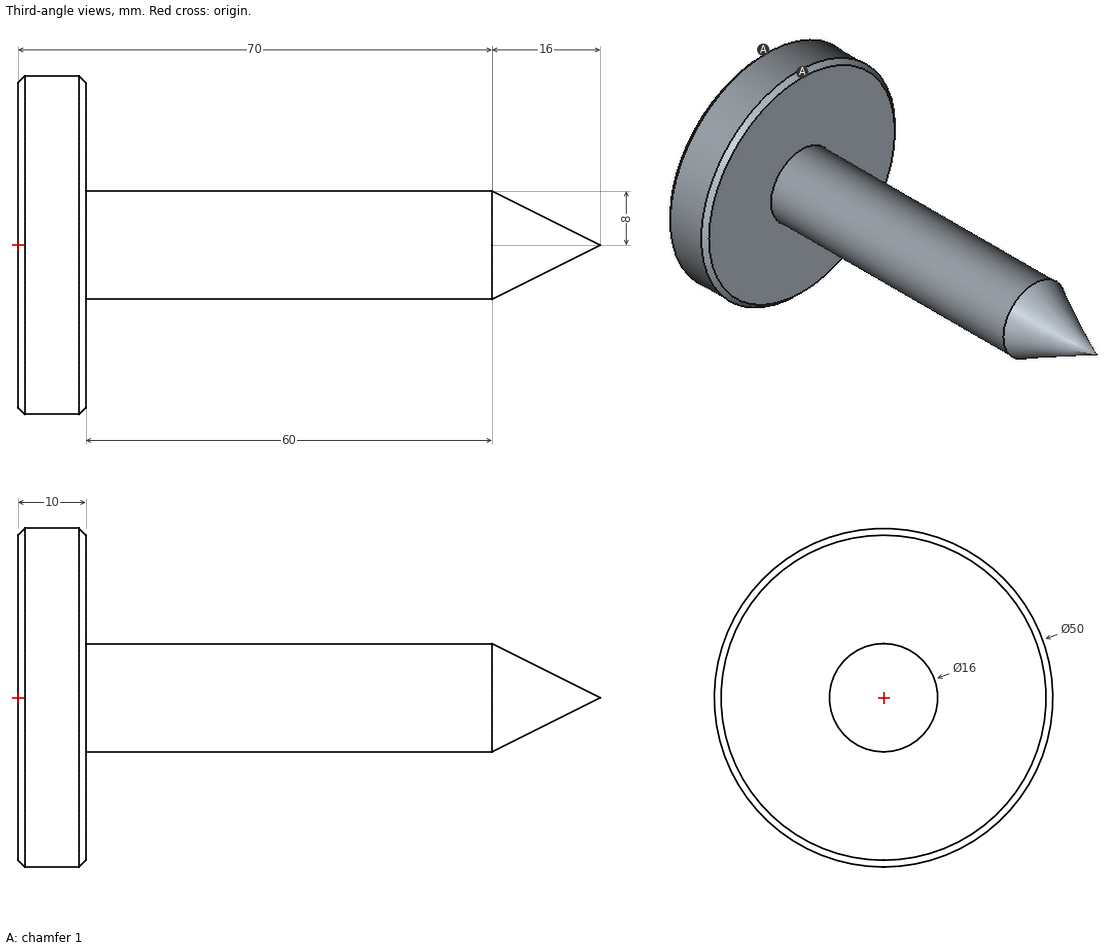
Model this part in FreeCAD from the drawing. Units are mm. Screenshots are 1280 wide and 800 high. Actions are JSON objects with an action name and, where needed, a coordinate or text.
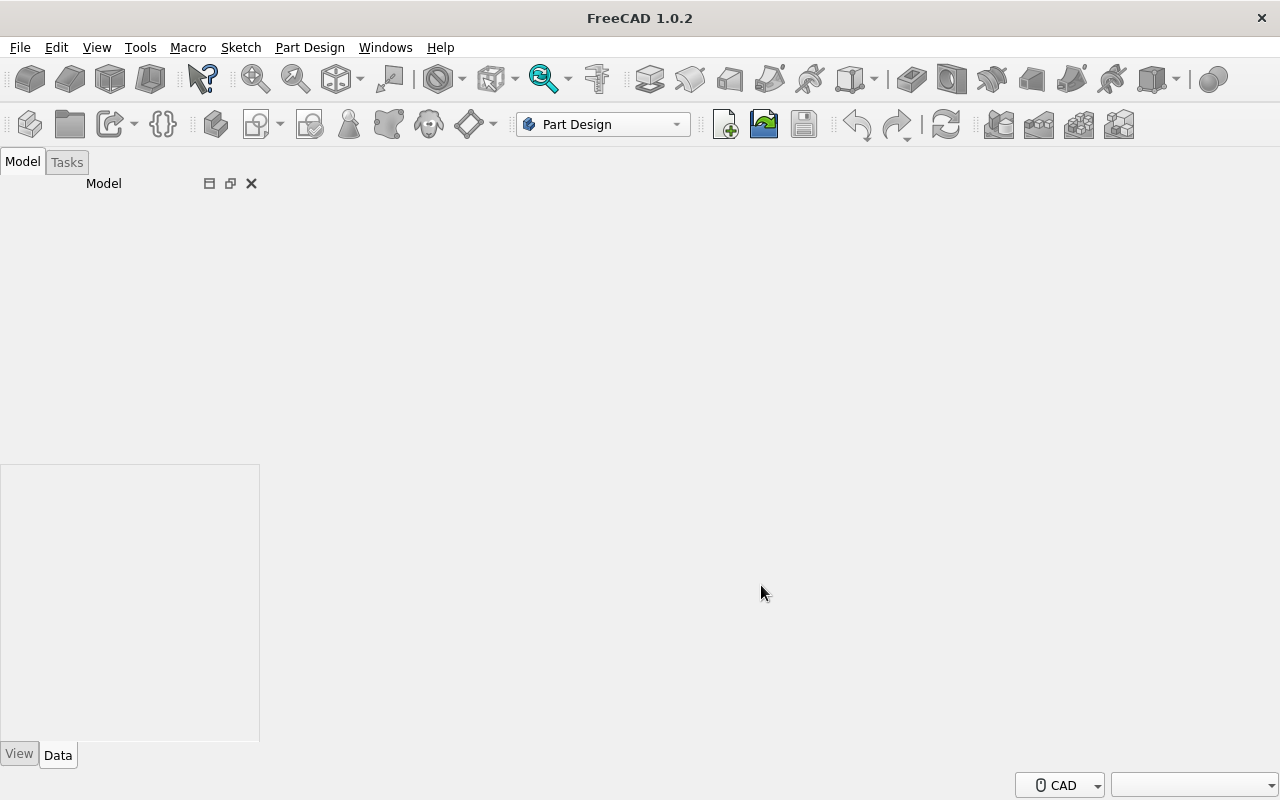
{"action": "left_click", "coordinate": [724, 124]}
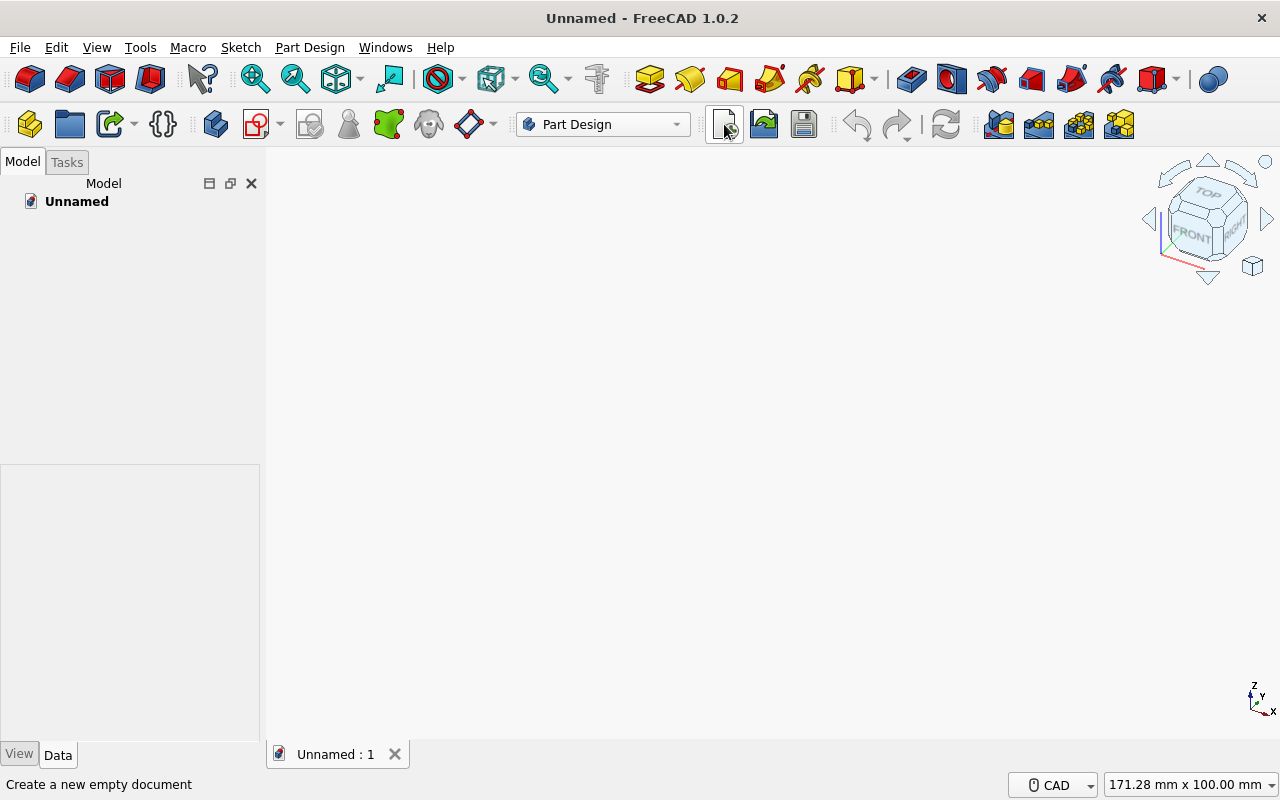
{"action": "left_click", "coordinate": [256, 124]}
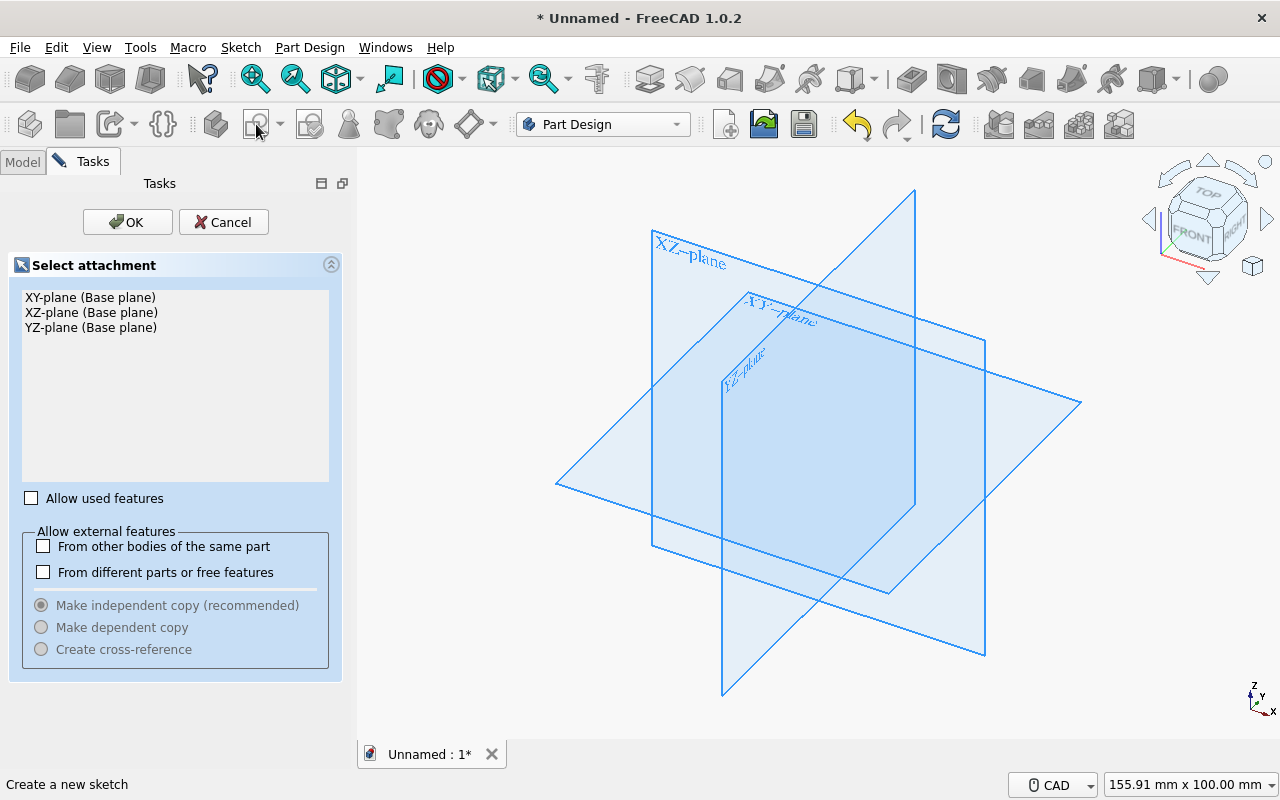
{"action": "left_click", "coordinate": [82, 328]}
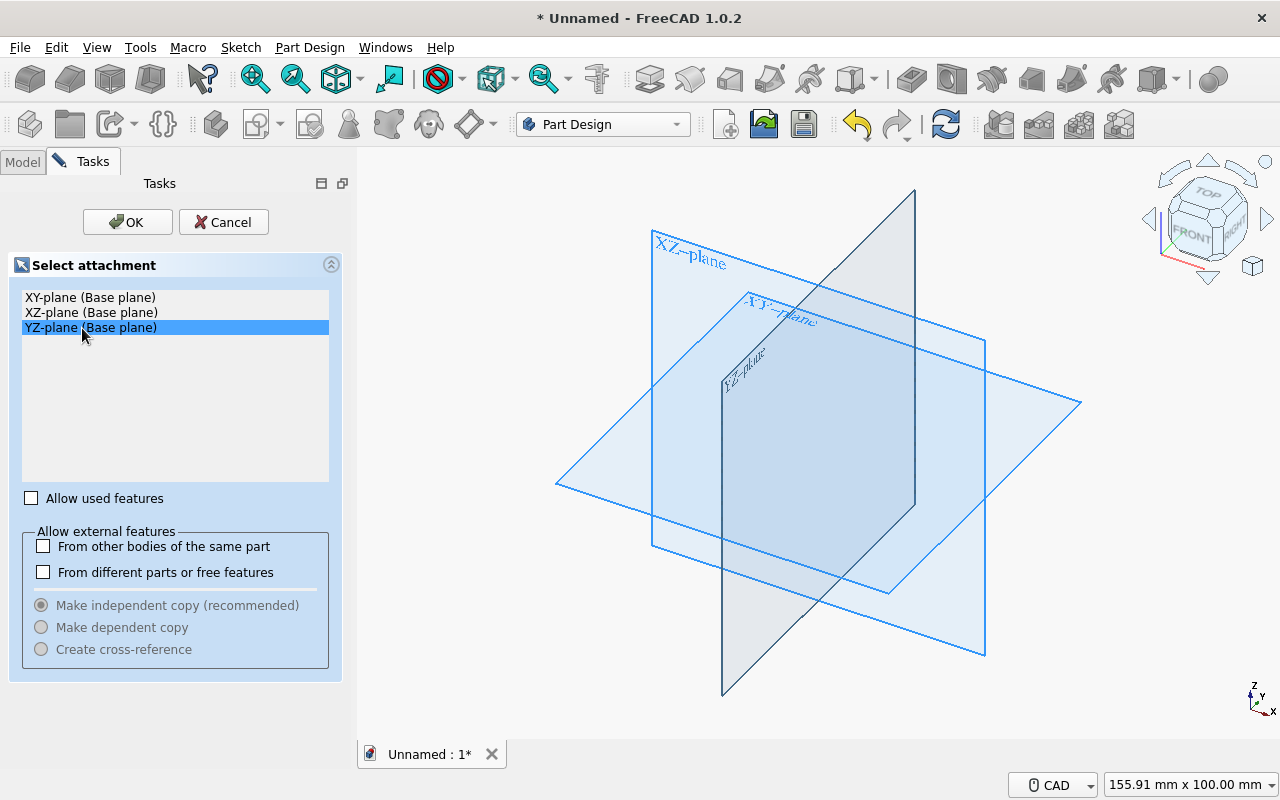
{"action": "left_click", "coordinate": [128, 222]}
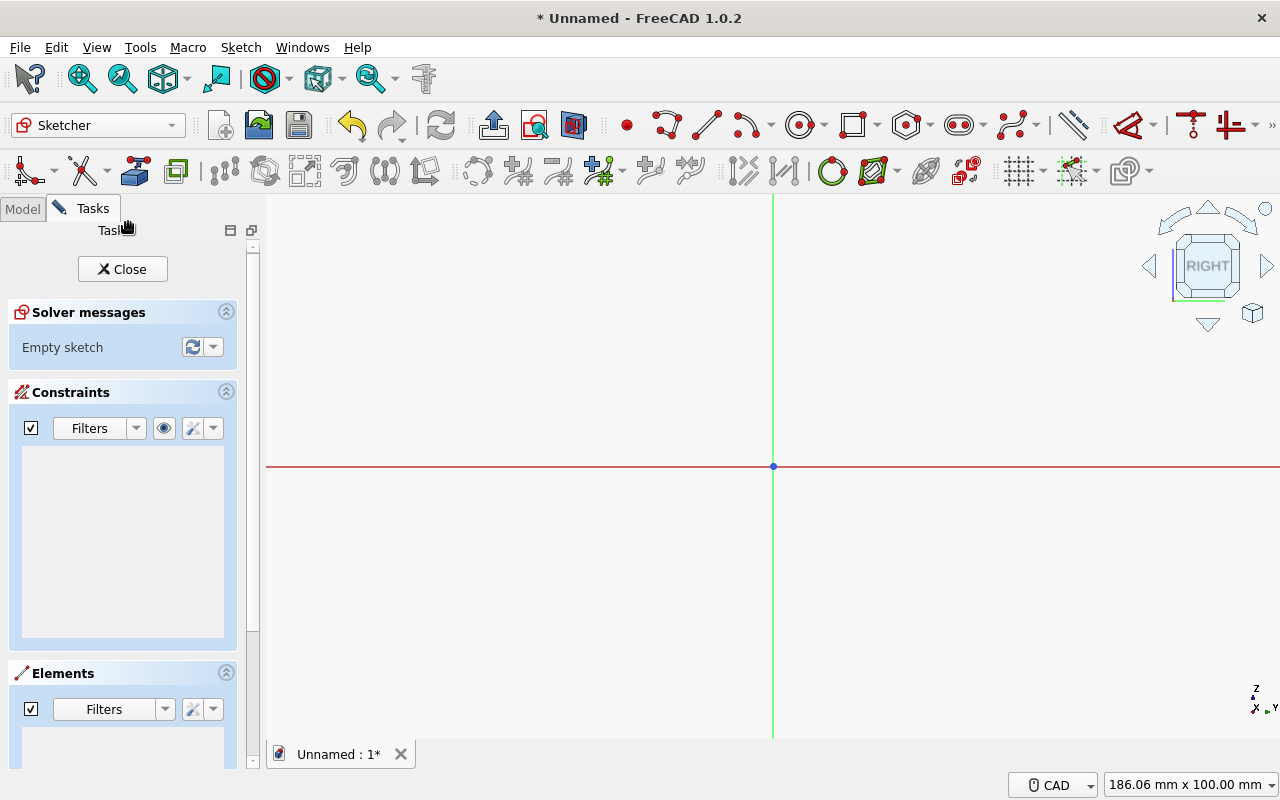
{"action": "left_click", "coordinate": [800, 126]}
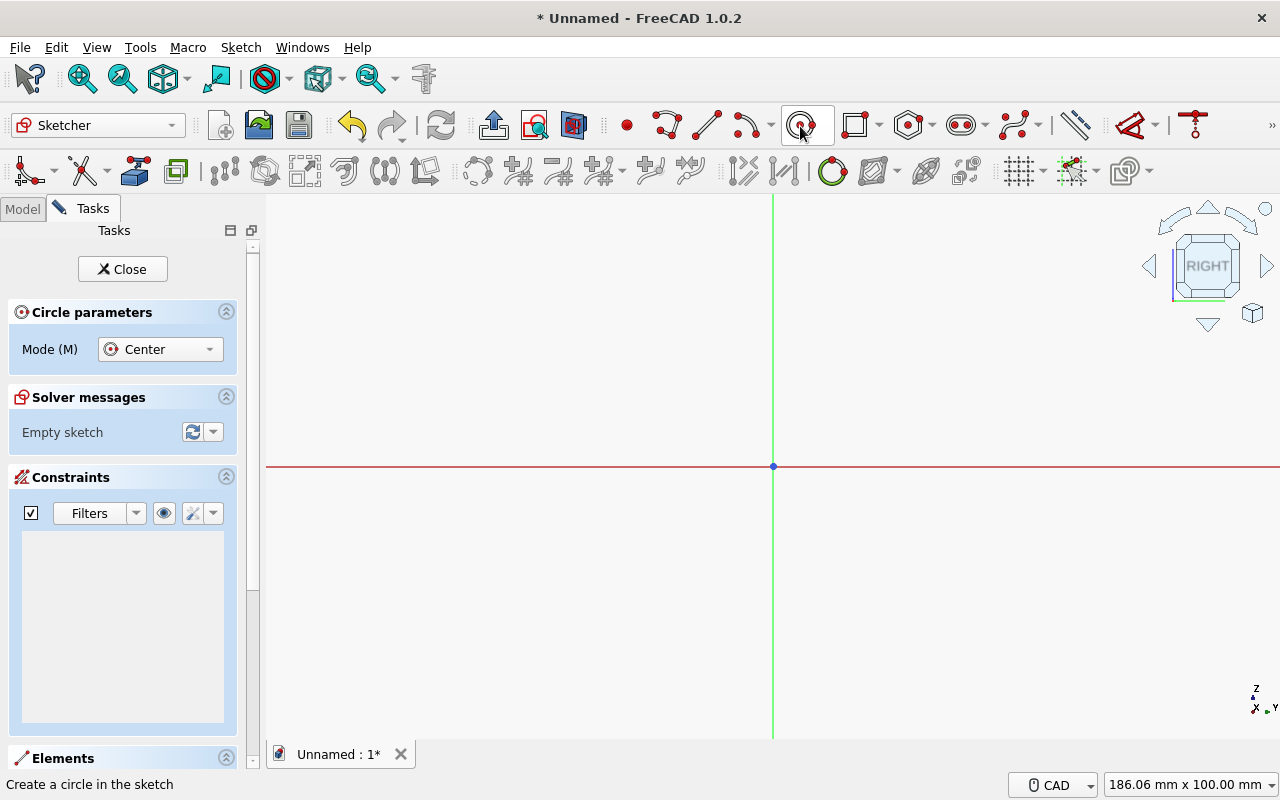
{"action": "left_click", "coordinate": [773, 466]}
{"action": "left_click", "coordinate": [869, 370]}
{"action": "key", "text": "Escape"}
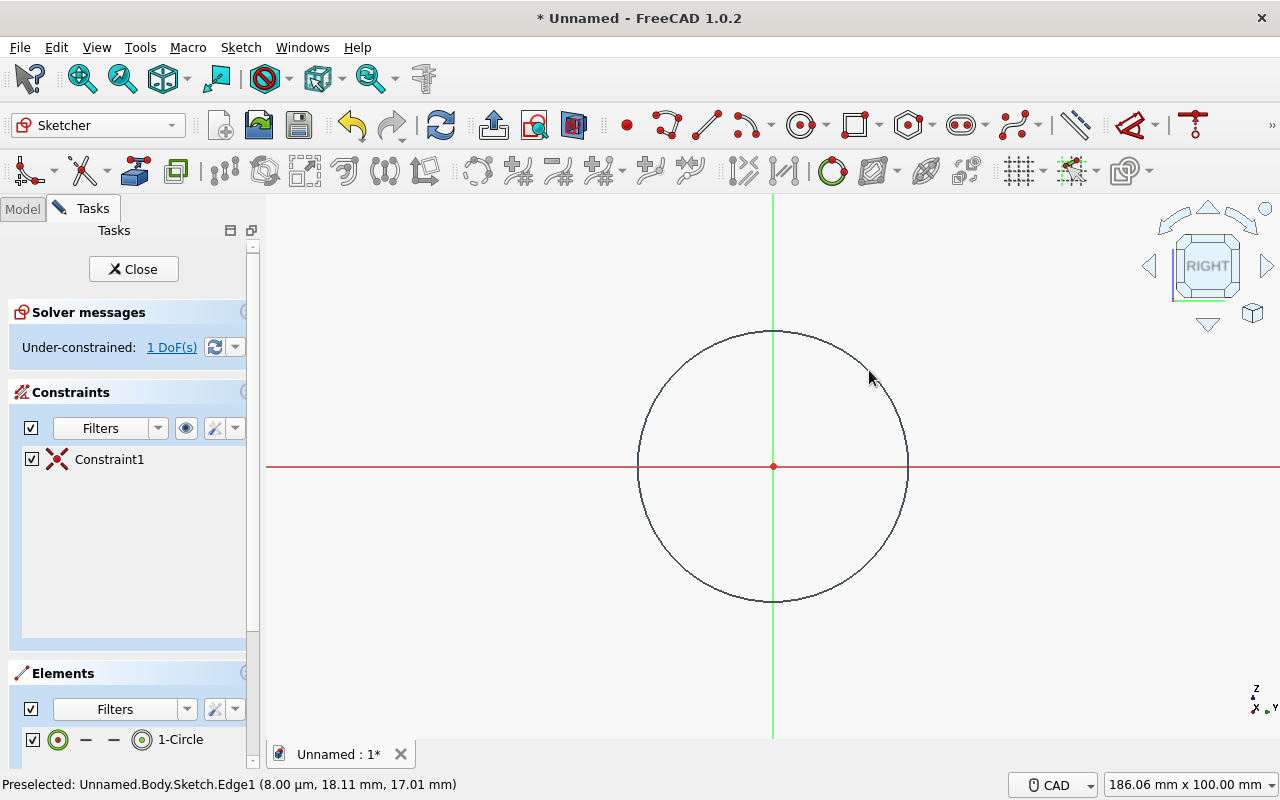
{"action": "left_click", "coordinate": [868, 370]}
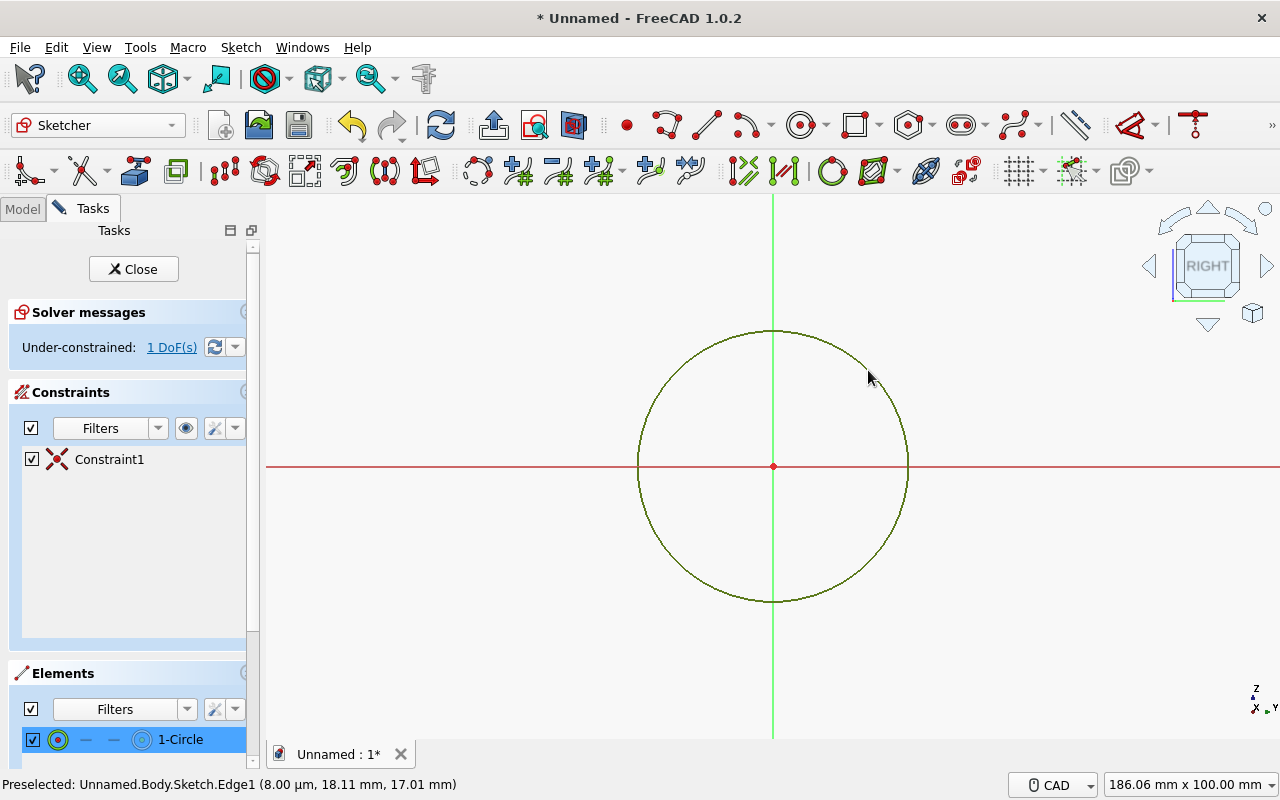
{"action": "left_click", "coordinate": [1158, 126]}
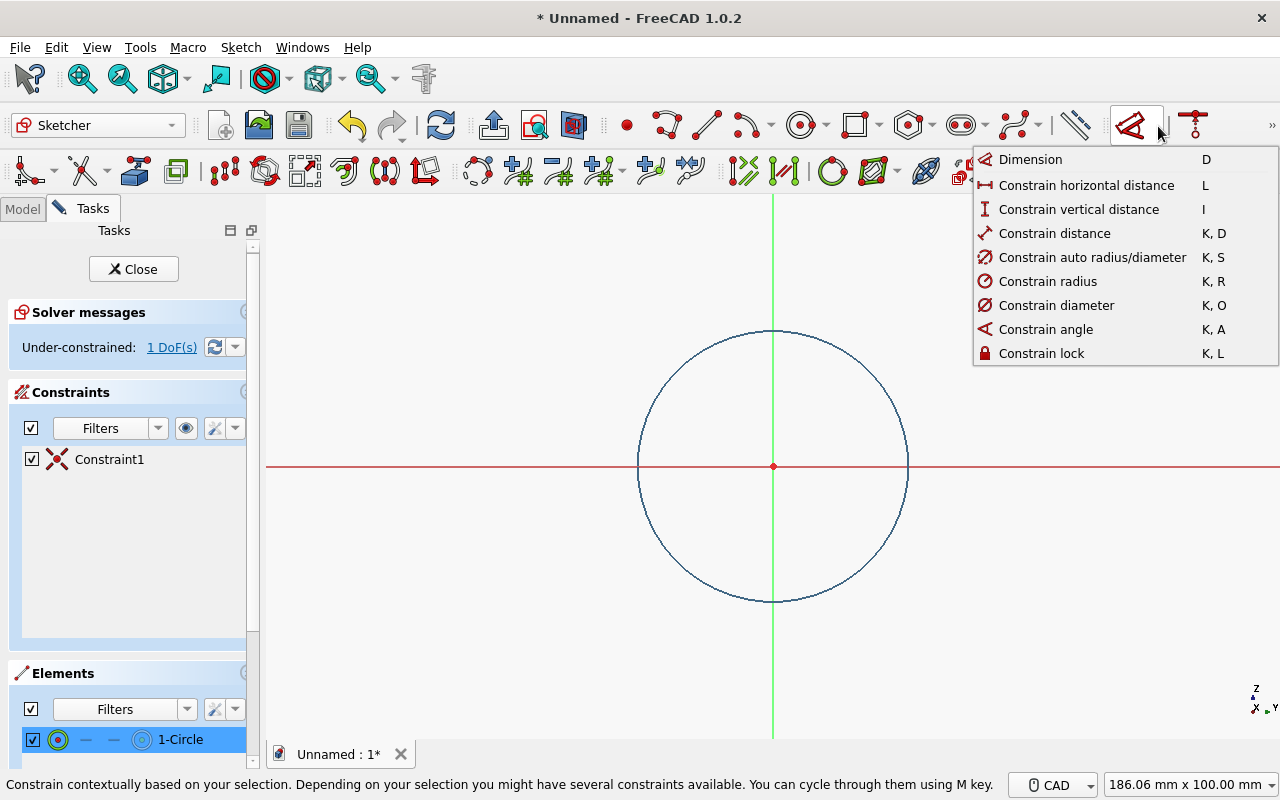
{"action": "left_click", "coordinate": [1126, 305]}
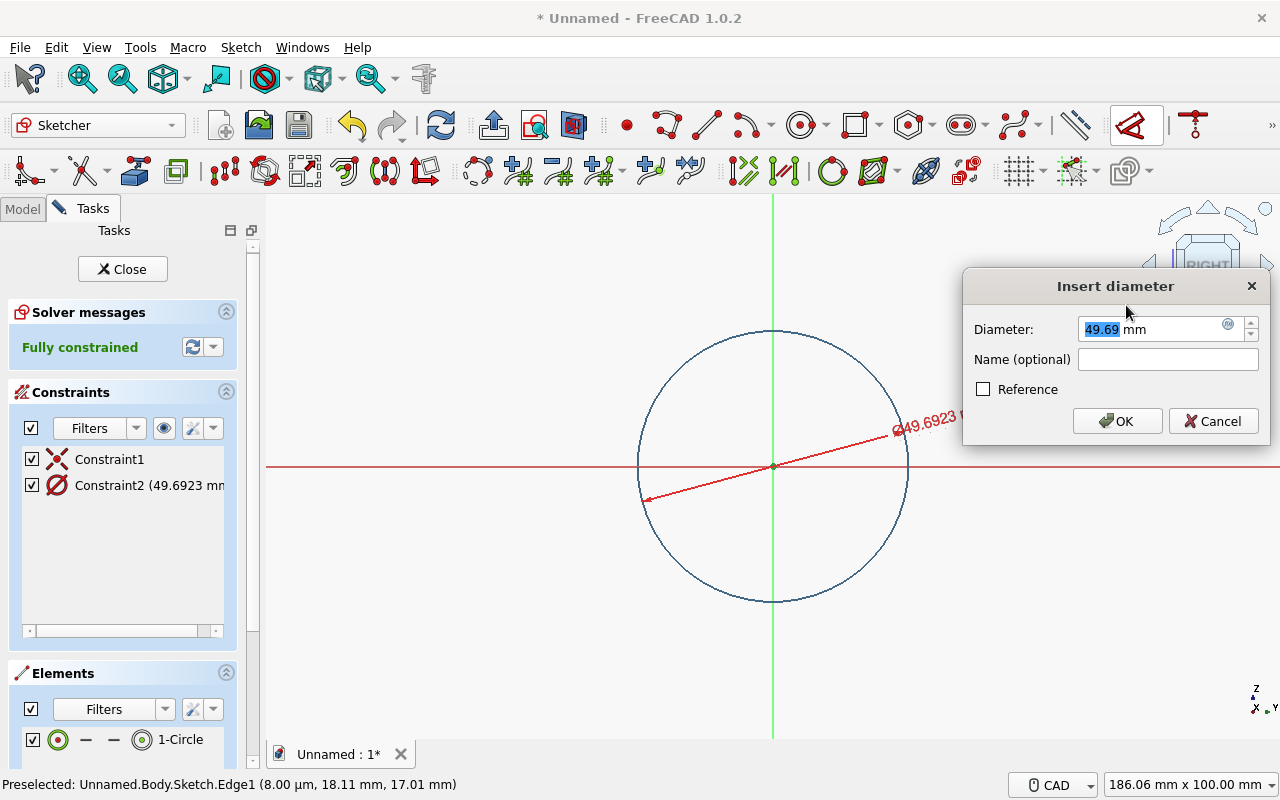
{"action": "type", "text": "50"}
{"action": "key", "text": "Return"}